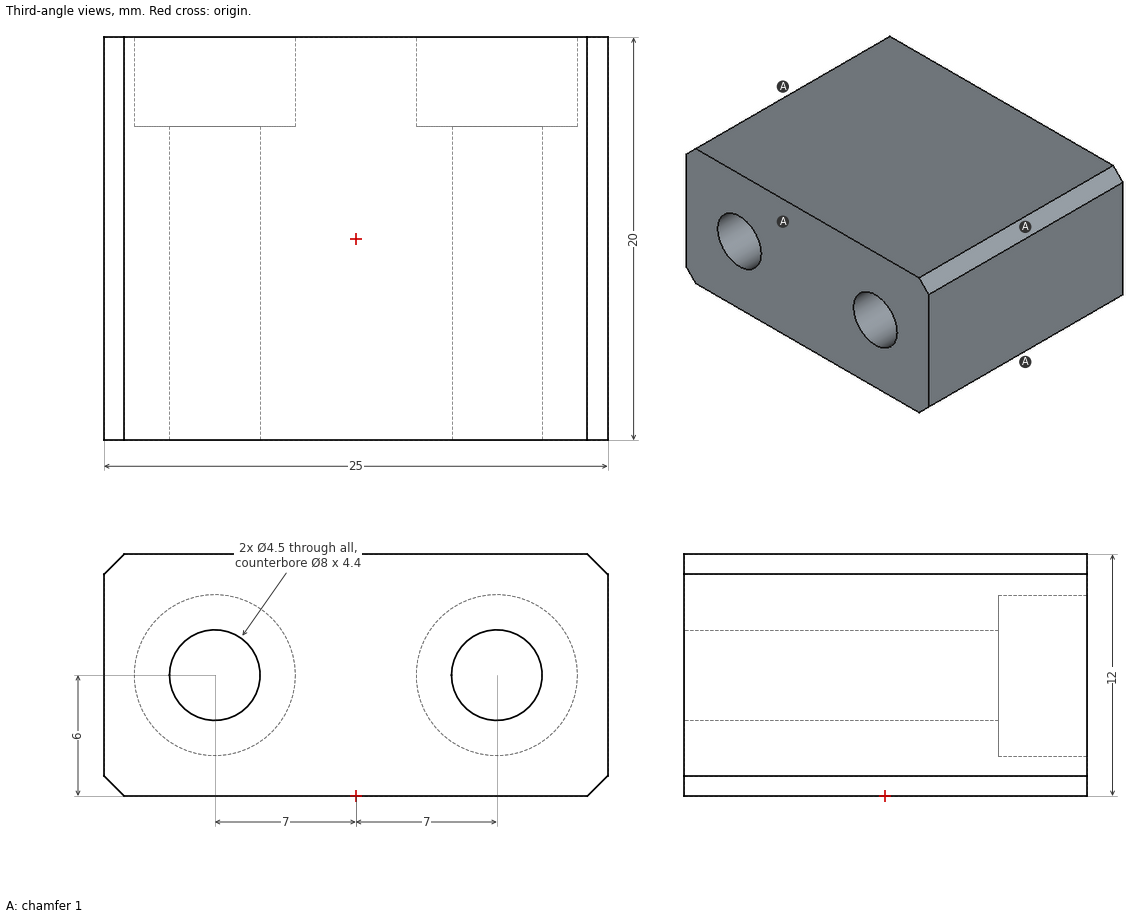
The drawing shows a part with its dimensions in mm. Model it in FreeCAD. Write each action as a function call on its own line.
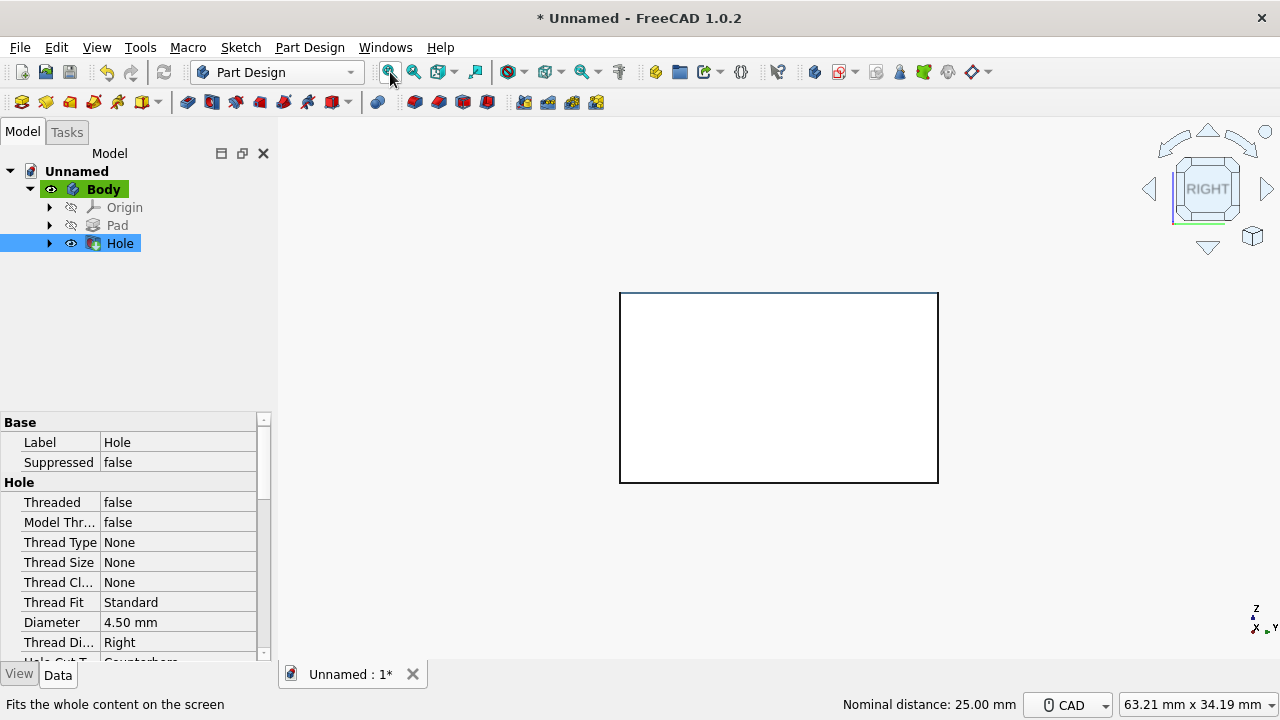
click(779, 482, ctrl)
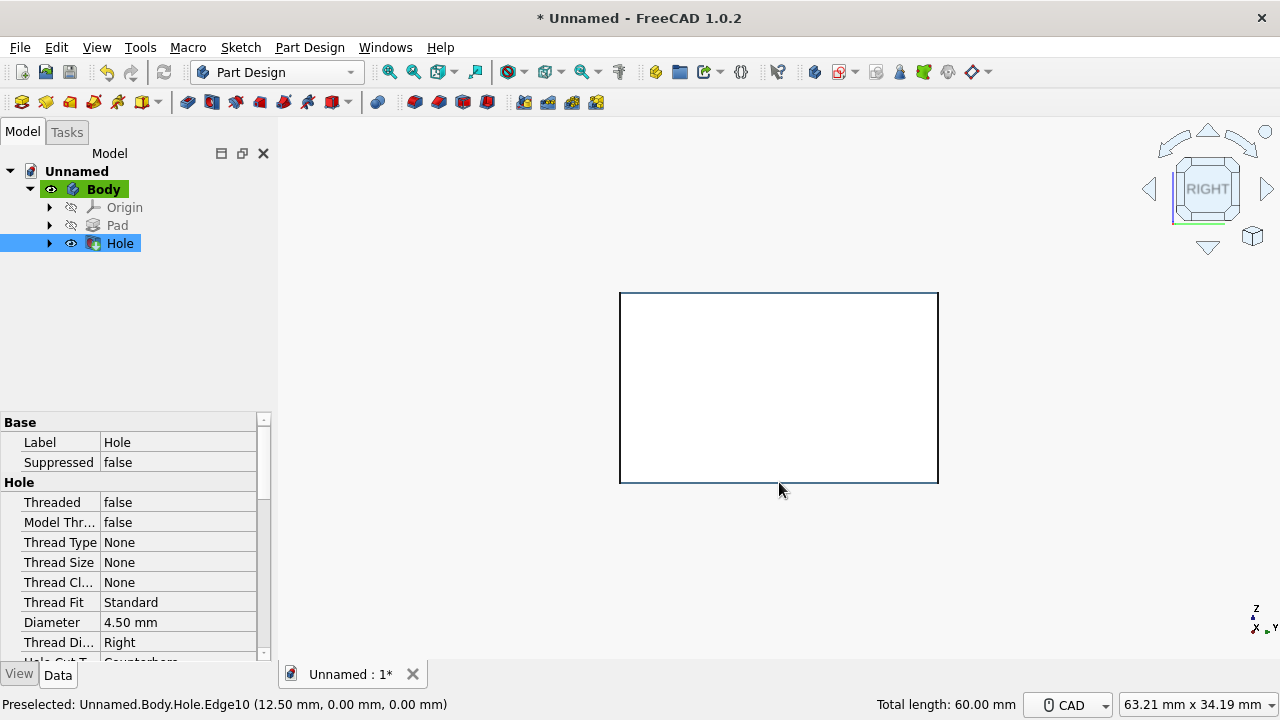
key(5)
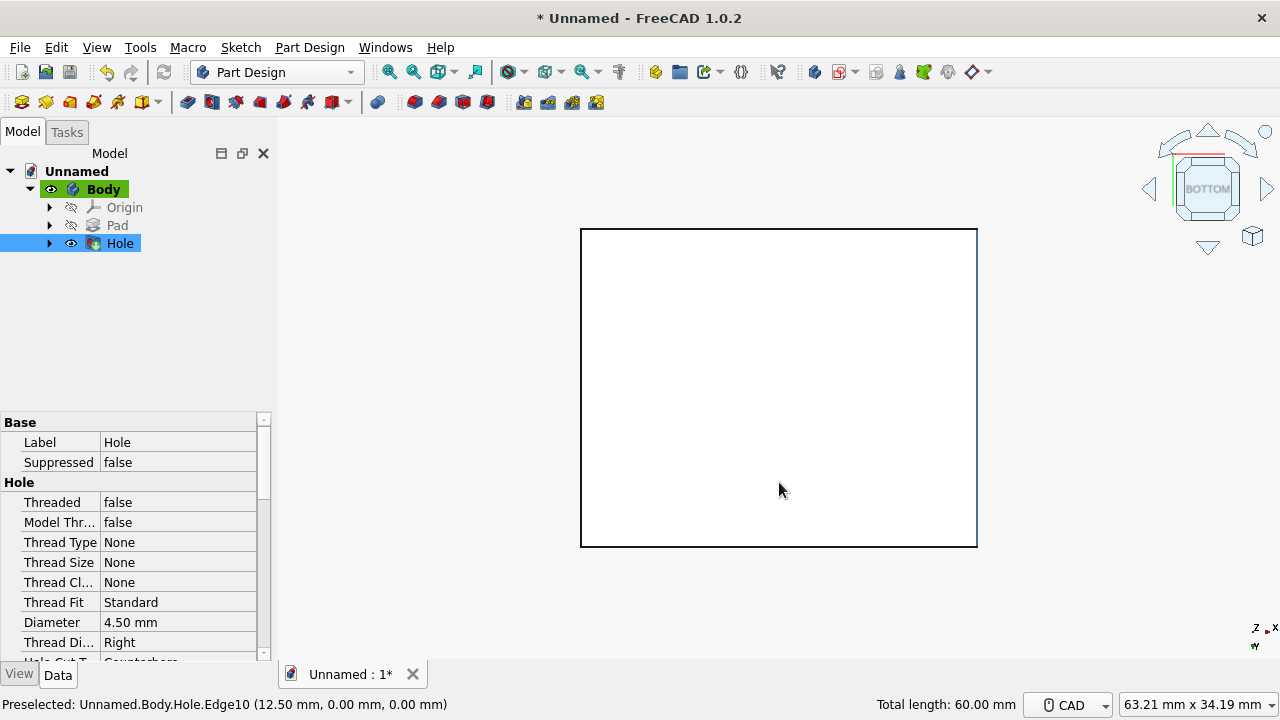
click(581, 387, ctrl)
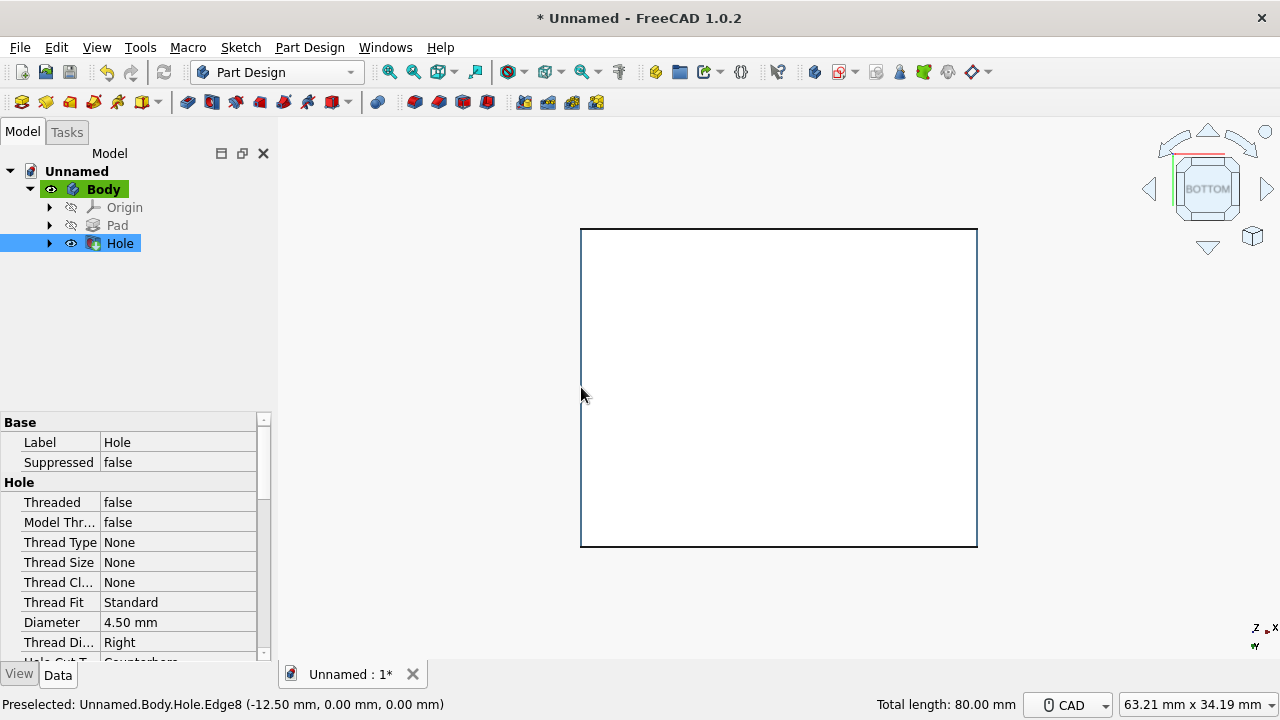
click(440, 102)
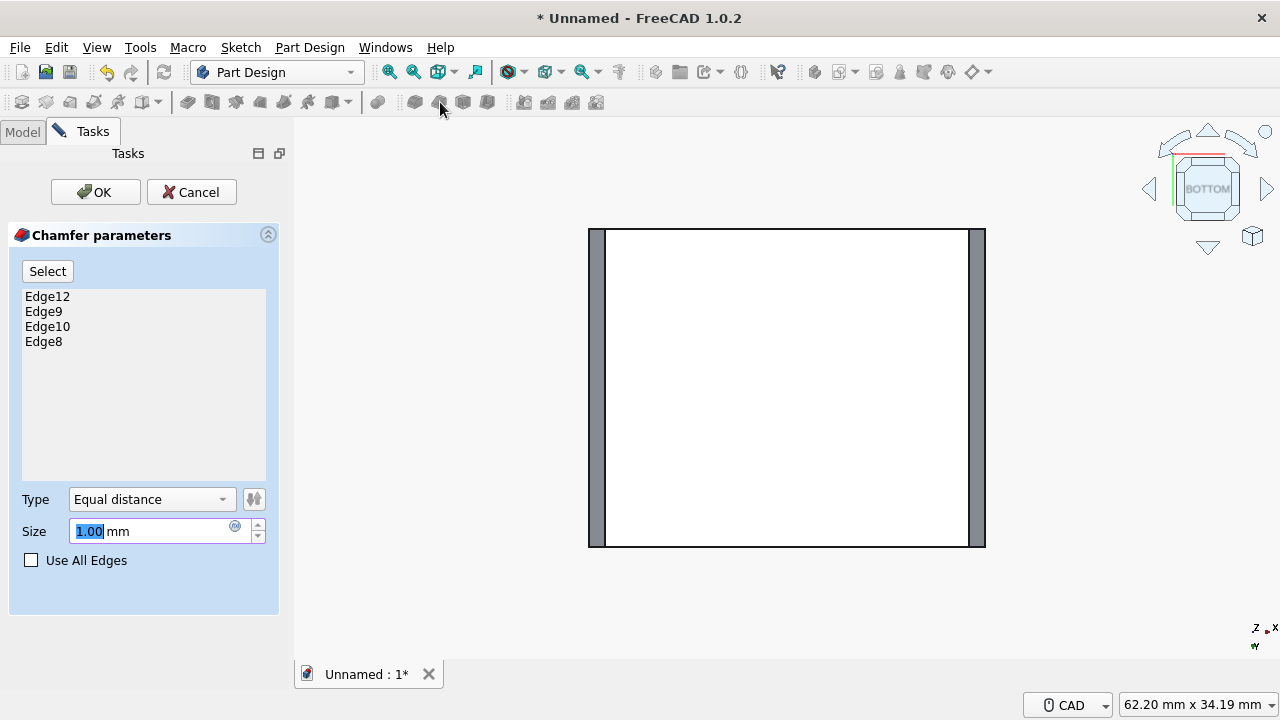
text(1)
key(Tab)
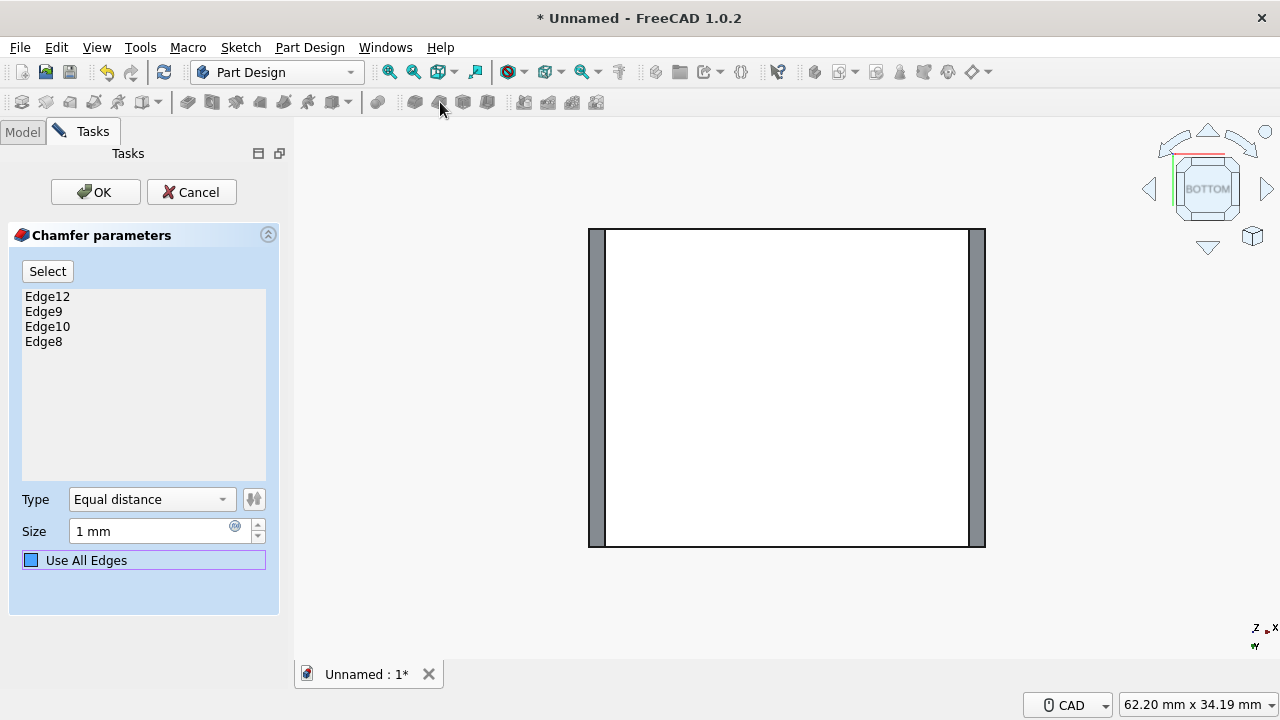
click(96, 192)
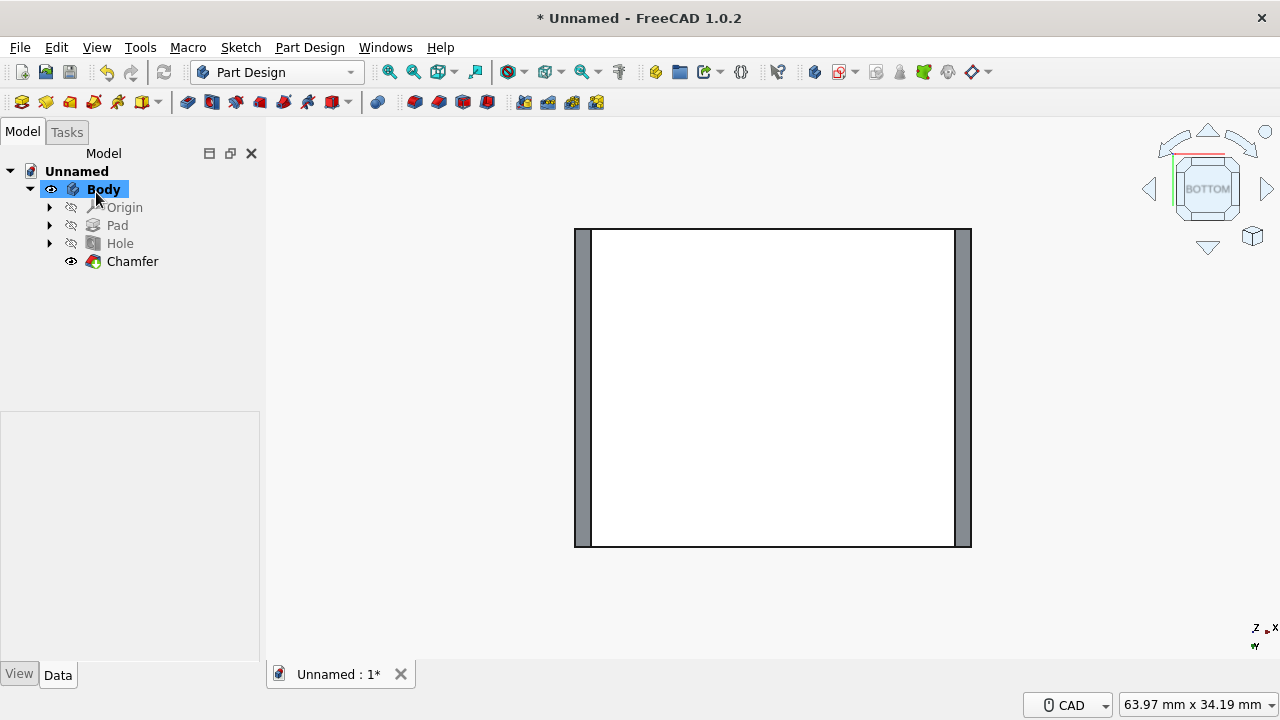
key(0)